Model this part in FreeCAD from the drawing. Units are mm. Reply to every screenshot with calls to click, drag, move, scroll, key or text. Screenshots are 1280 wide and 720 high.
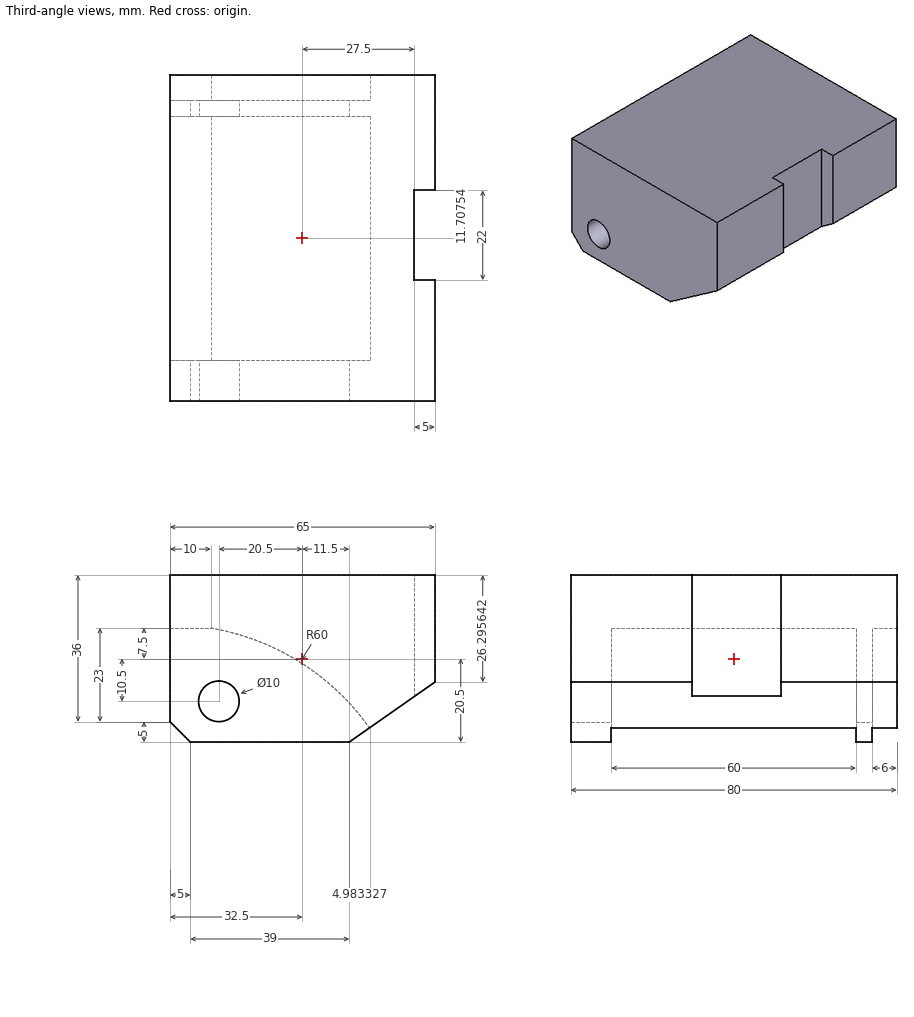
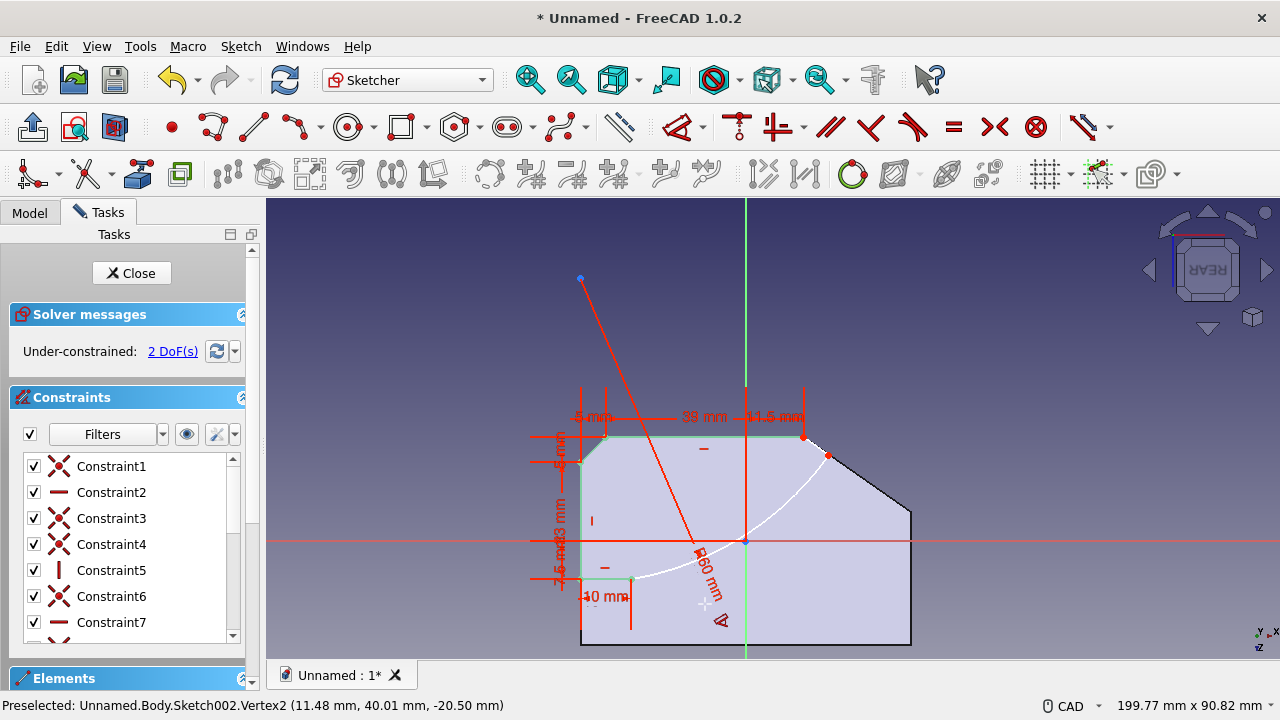
click(580, 279)
click(663, 245)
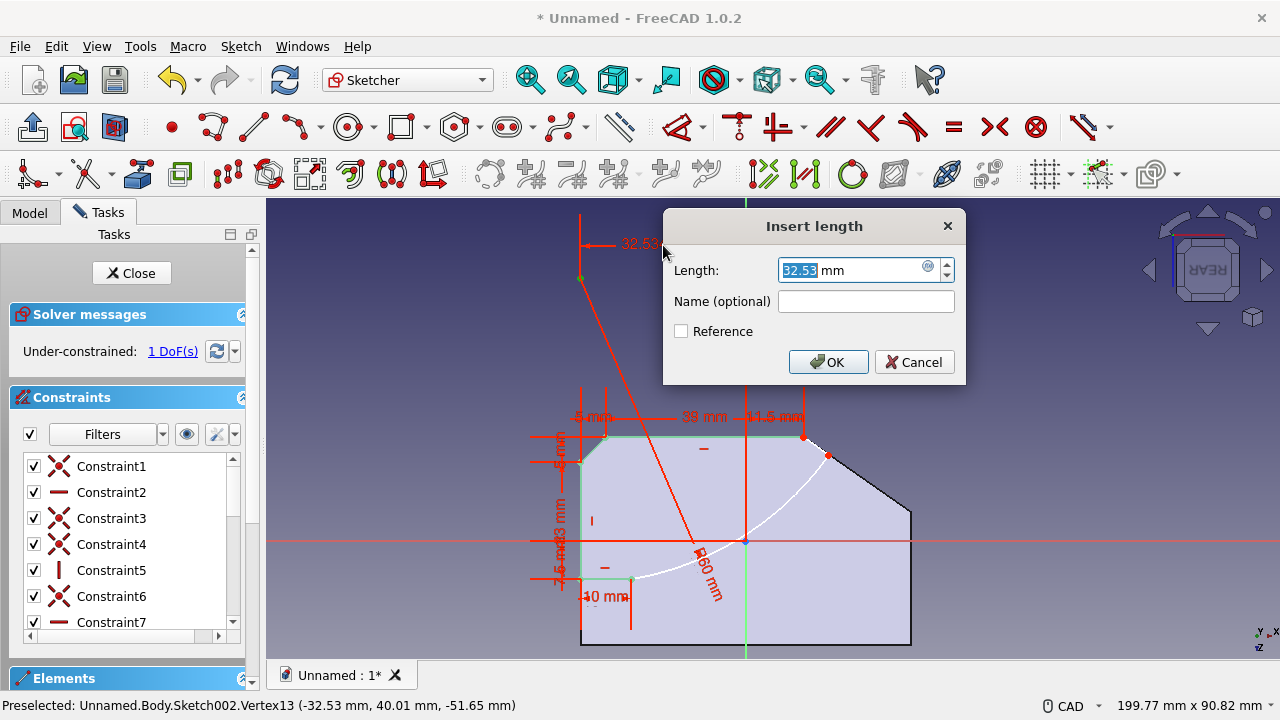
text(32.5)
key(Return)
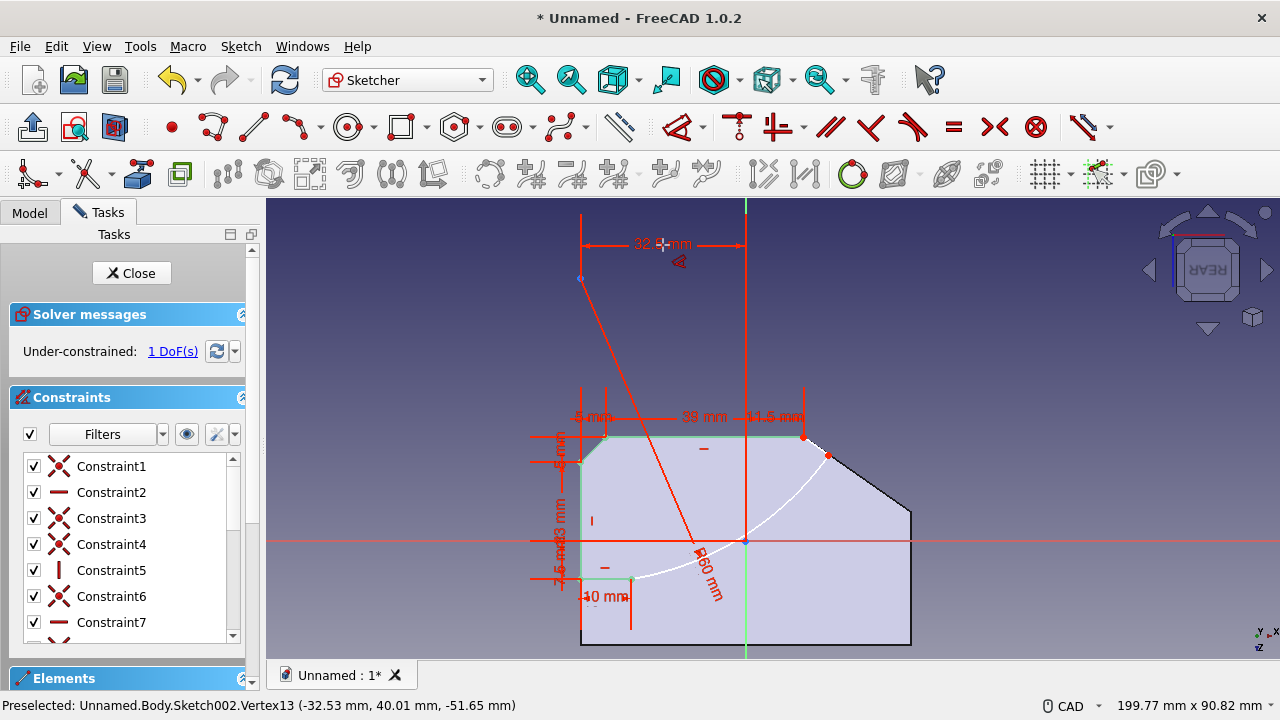
scroll(821, 450, up, 3)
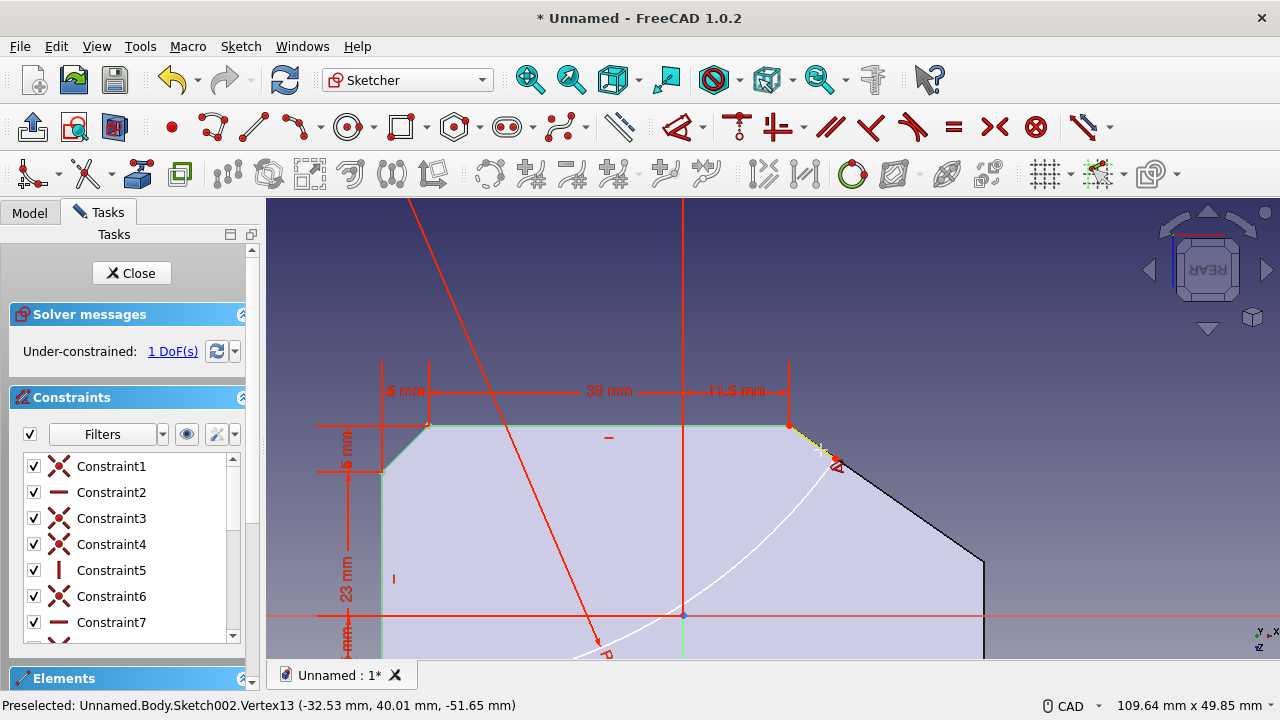
click(821, 449)
click(812, 392)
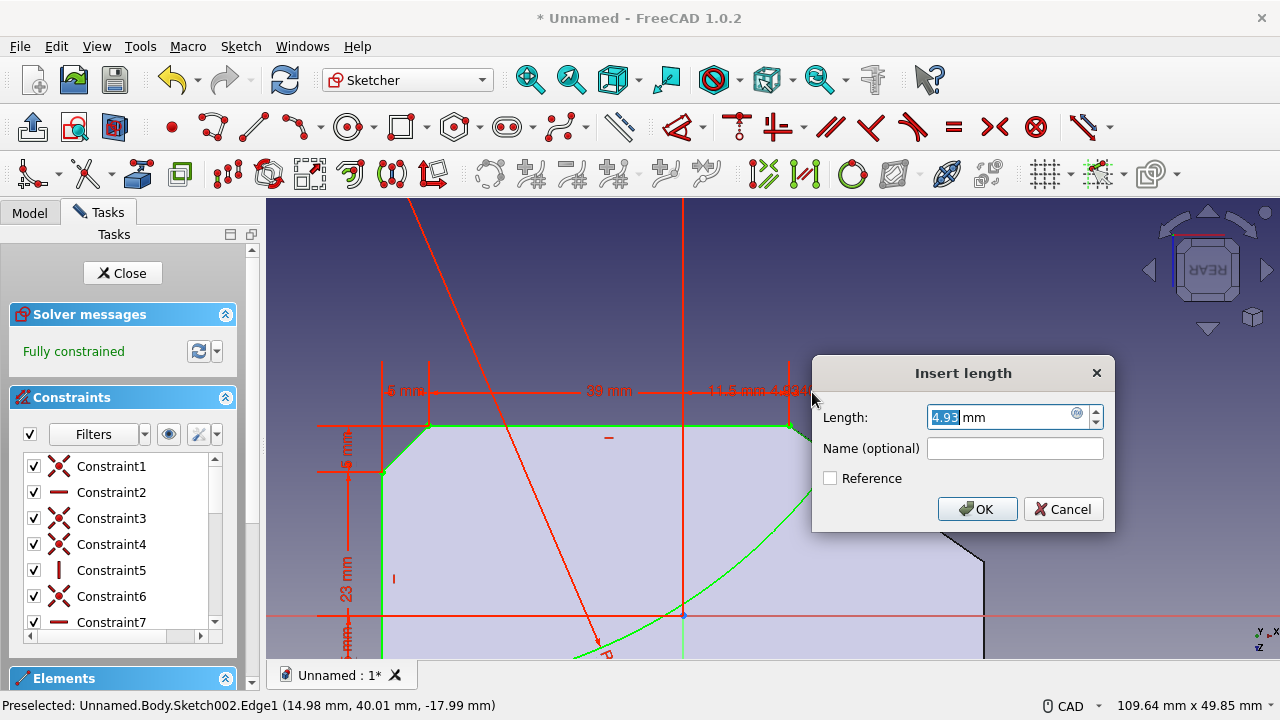
text(4.983327)
key(Return)
key(Escape)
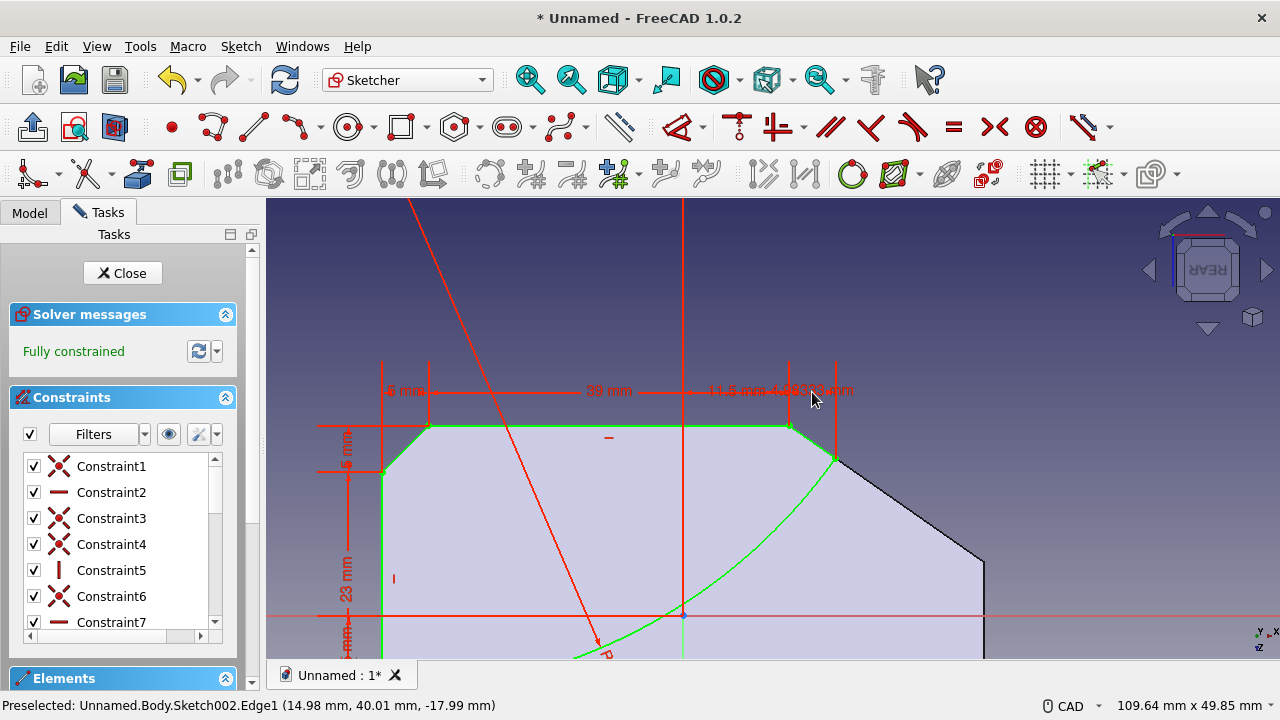
click(123, 273)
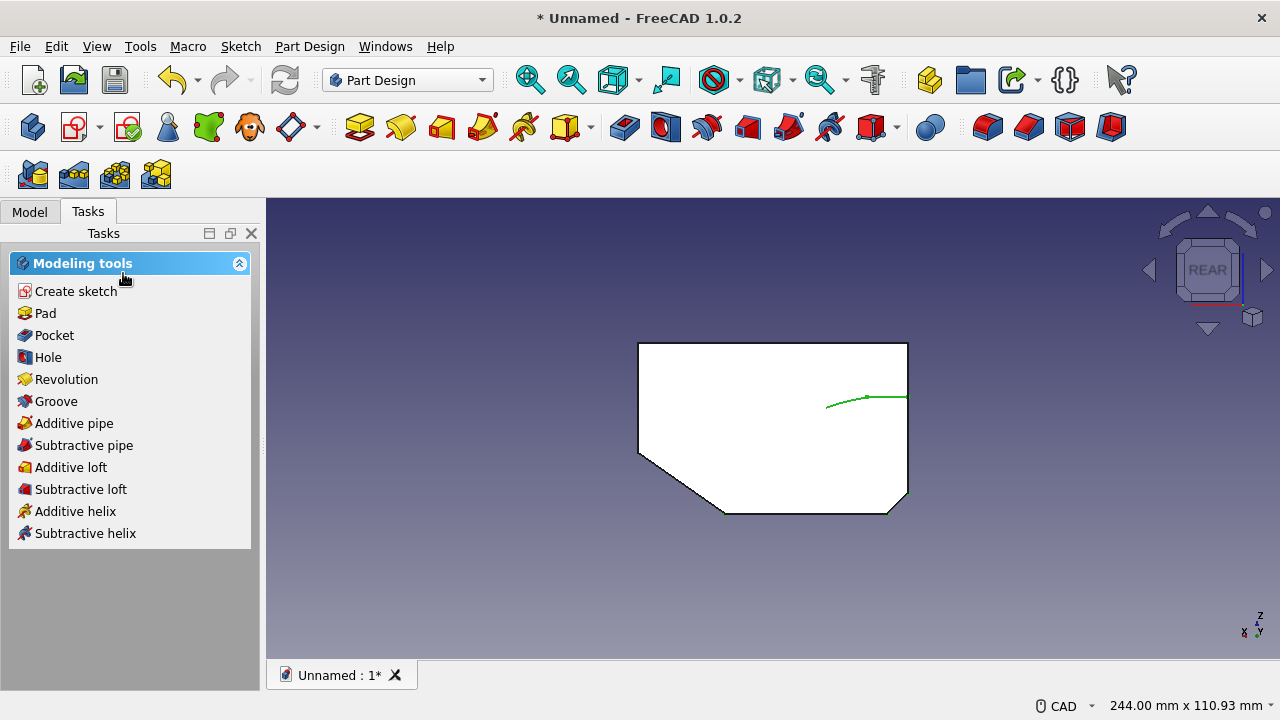
click(625, 128)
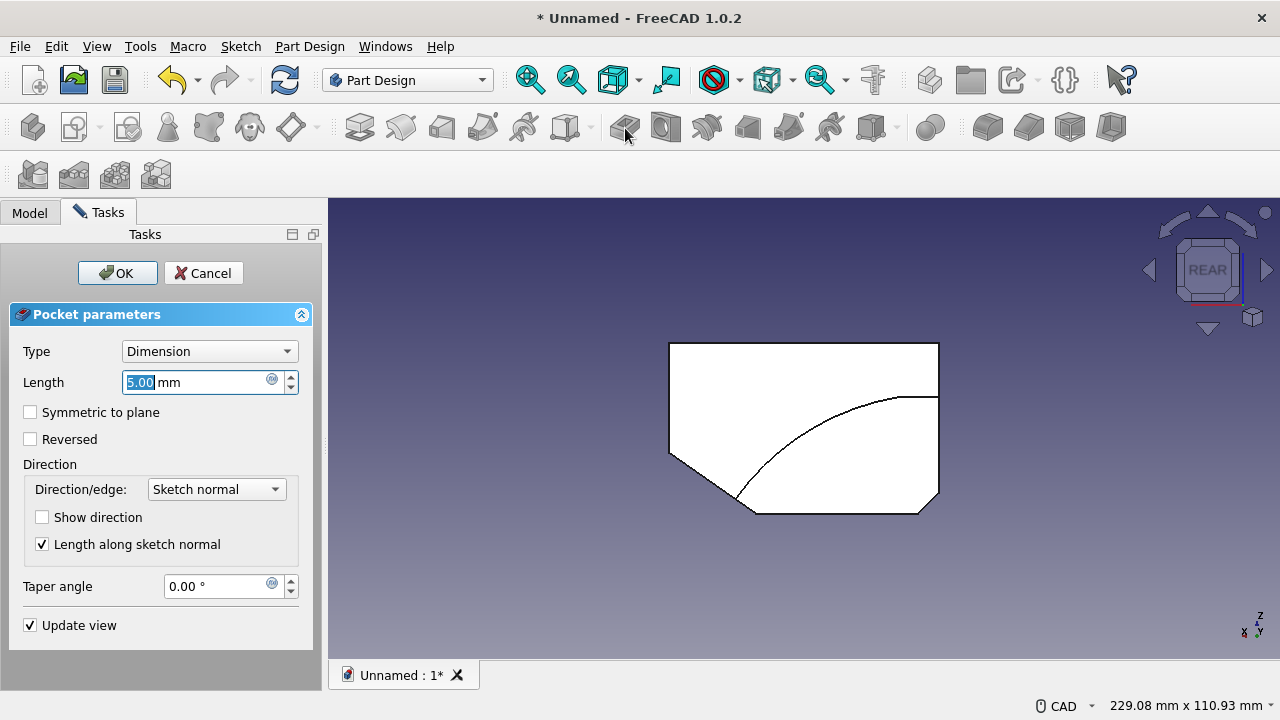
text(6)
key(Tab)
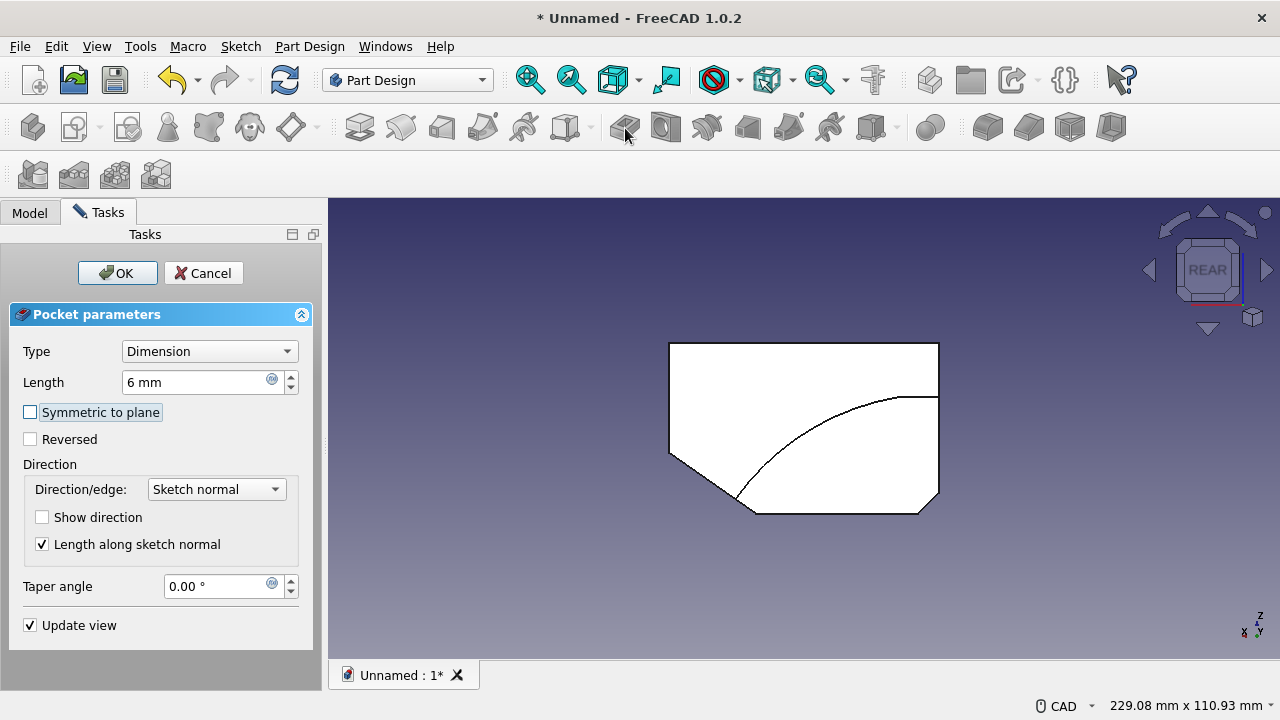
click(118, 273)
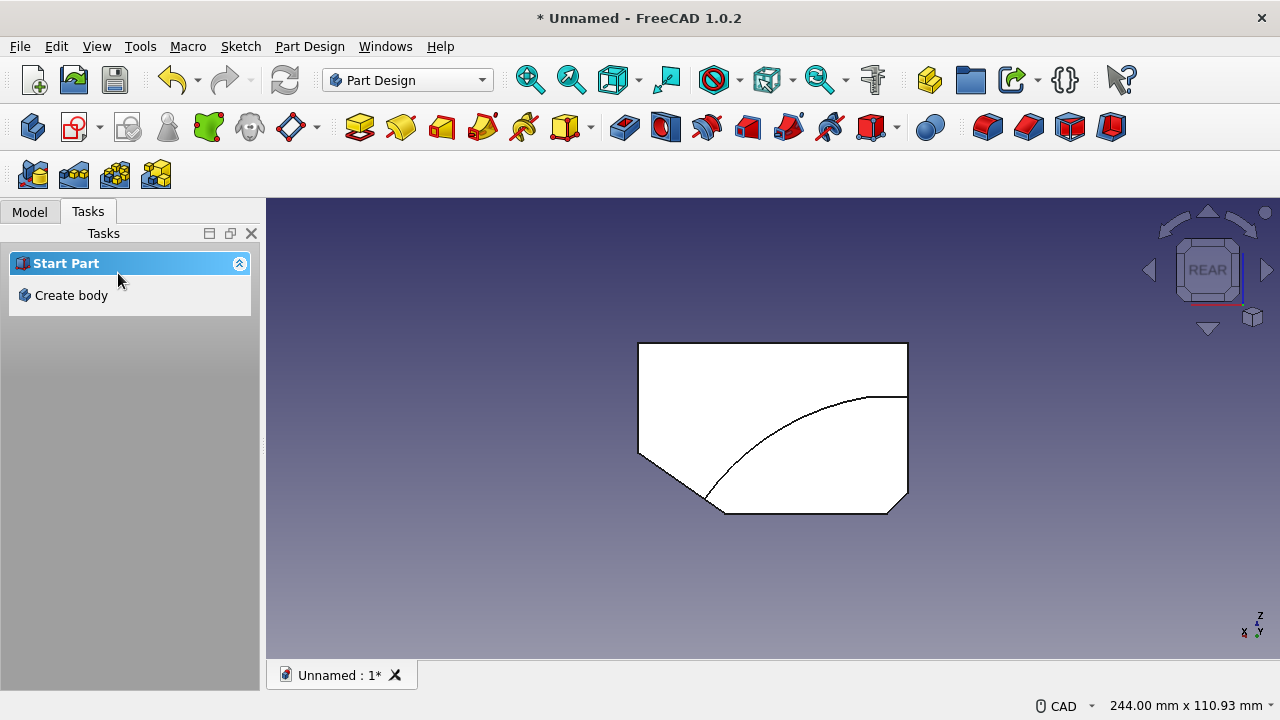
key(v)
key(f)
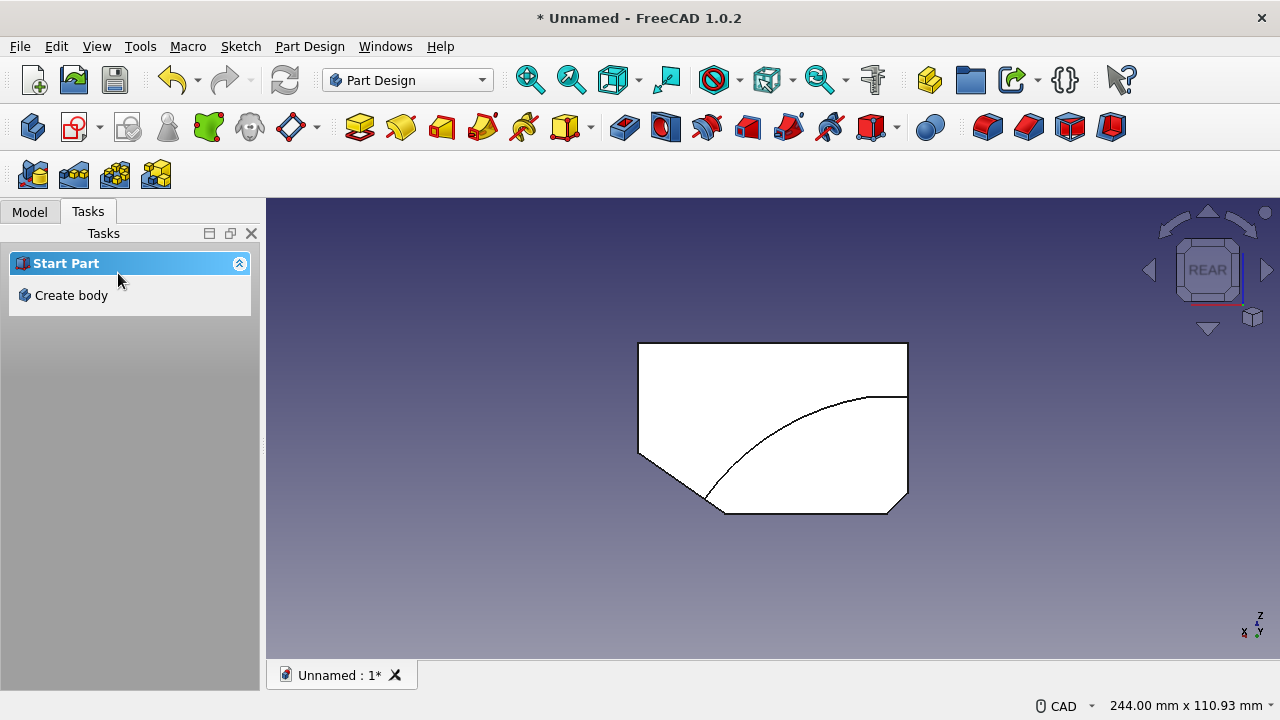
click(74, 128)